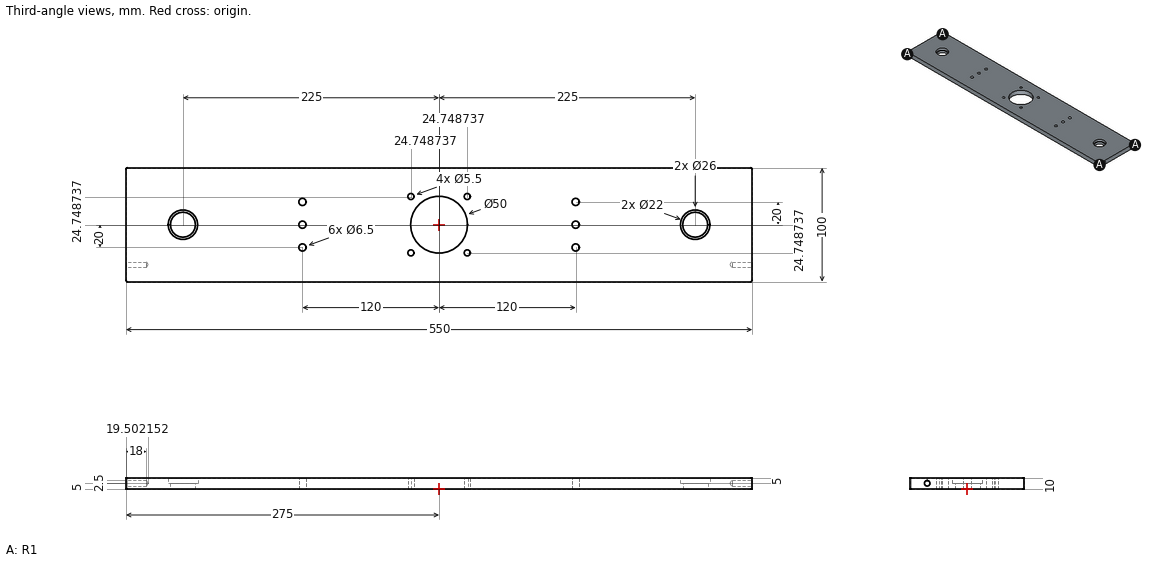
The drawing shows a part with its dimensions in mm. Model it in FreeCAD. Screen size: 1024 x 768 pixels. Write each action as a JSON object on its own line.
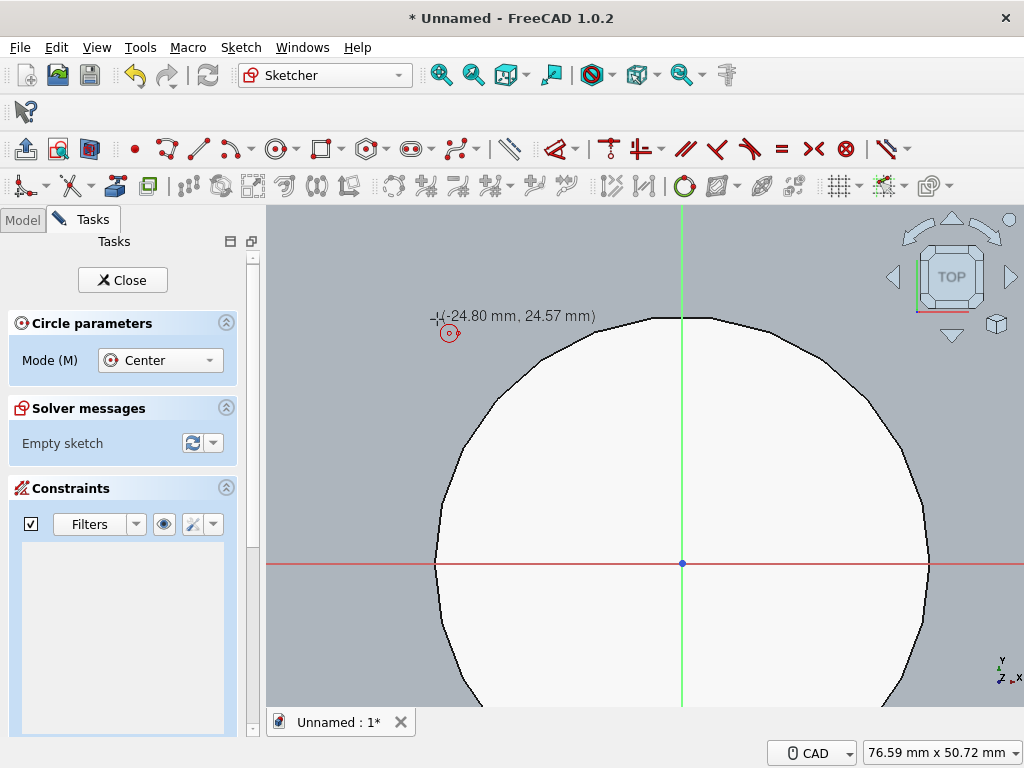
{"action": "left_click", "coordinate": [437, 319]}
{"action": "left_click", "coordinate": [457, 300]}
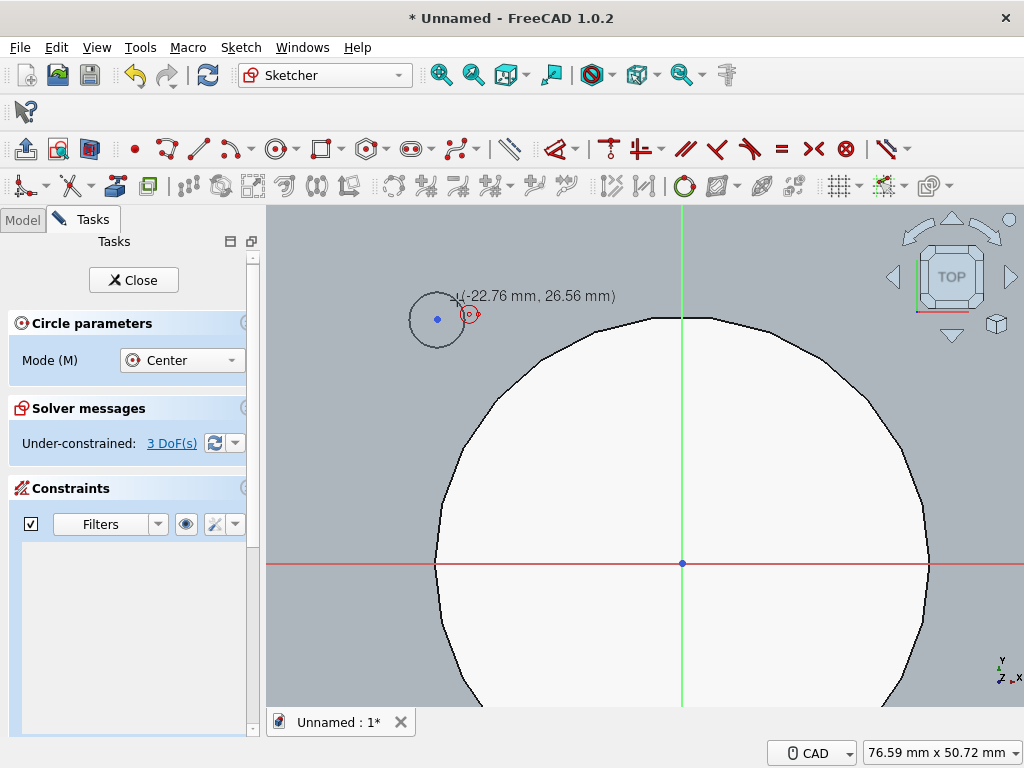
{"action": "scroll", "coordinate": [448, 325], "scroll_direction": "down", "scroll_amount": 3}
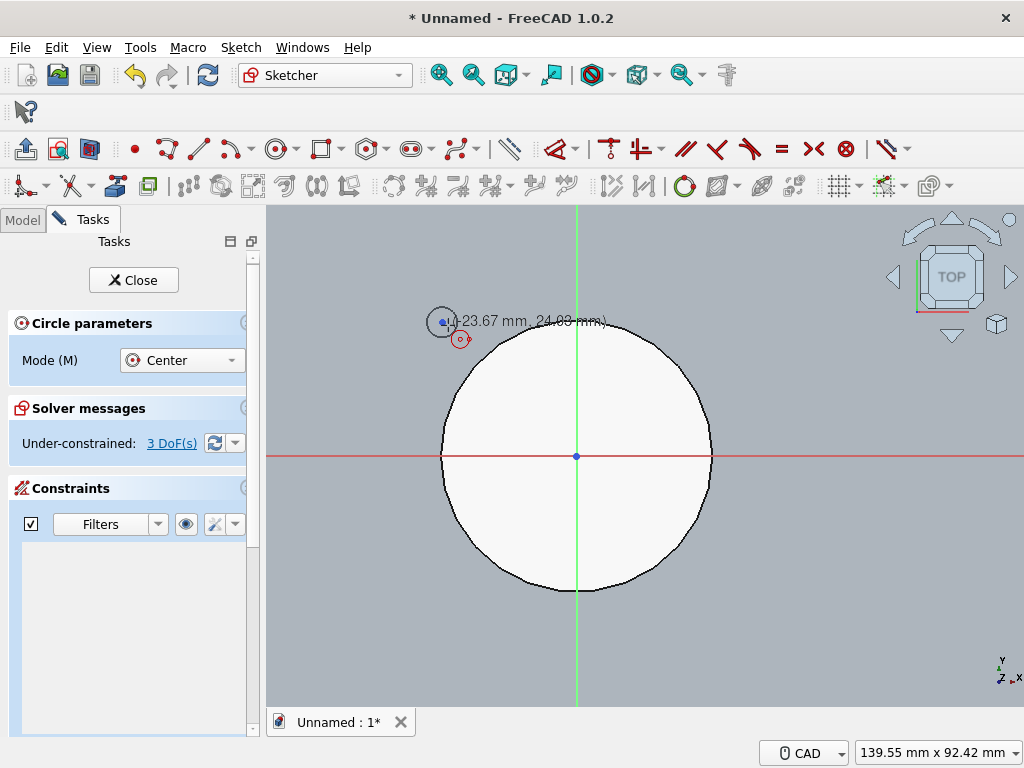
{"action": "scroll", "coordinate": [711, 322], "scroll_direction": "up", "scroll_amount": 3}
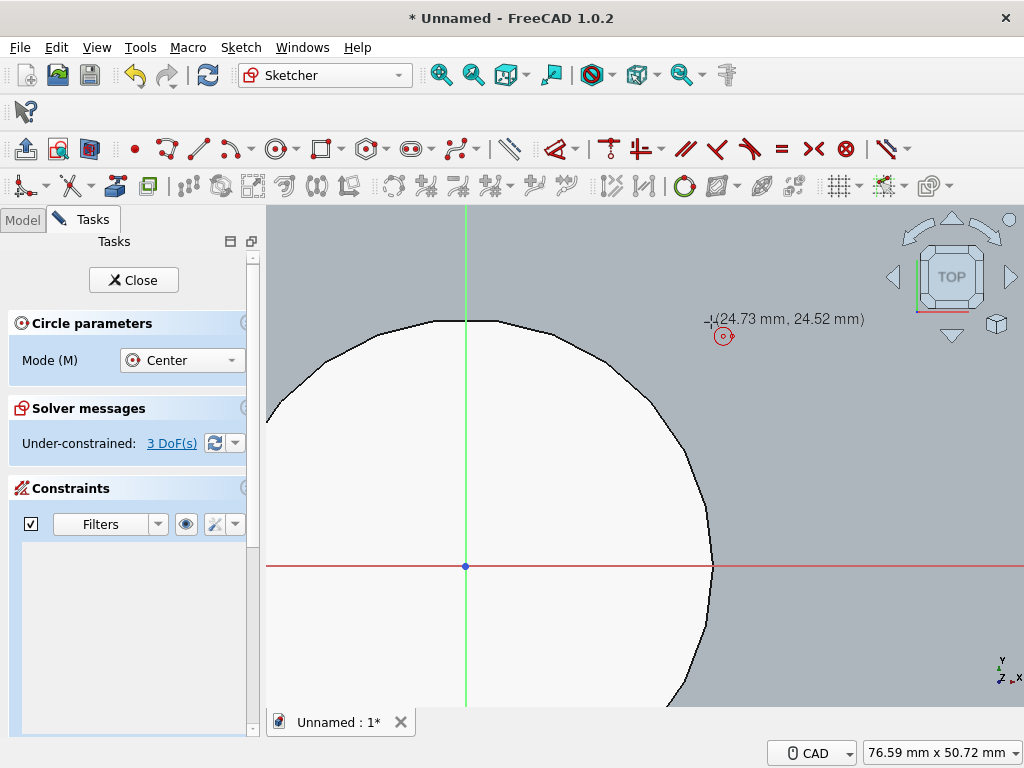
{"action": "left_click", "coordinate": [711, 321]}
{"action": "left_click", "coordinate": [730, 302]}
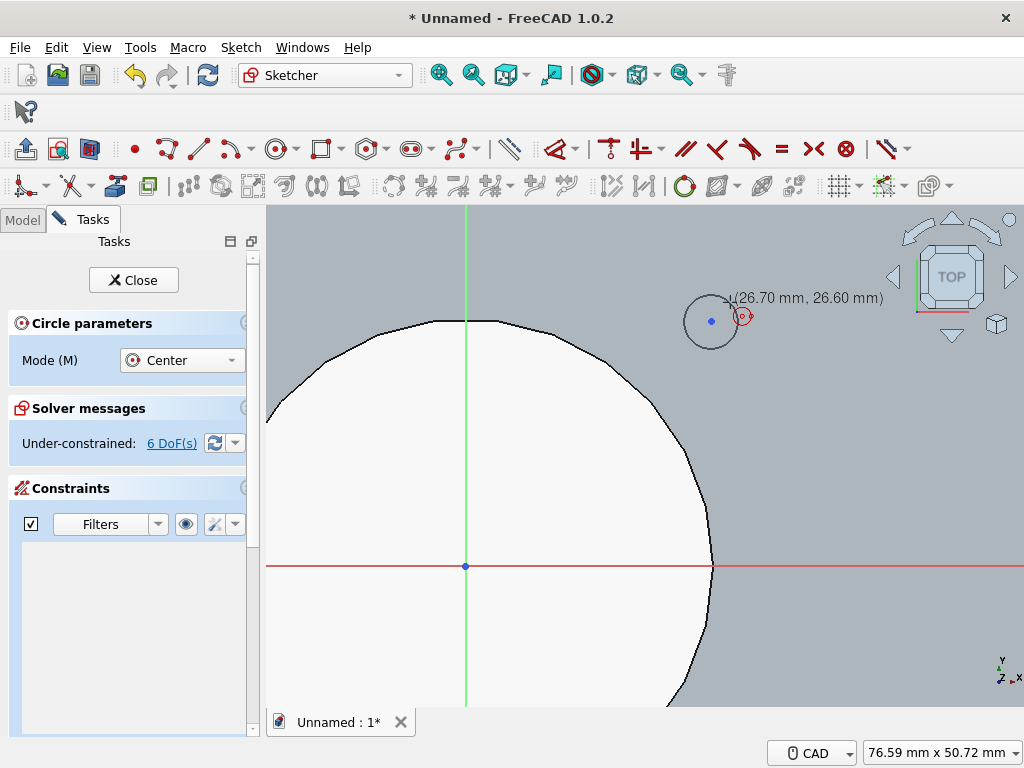
{"action": "scroll", "coordinate": [711, 322], "scroll_direction": "down", "scroll_amount": 3}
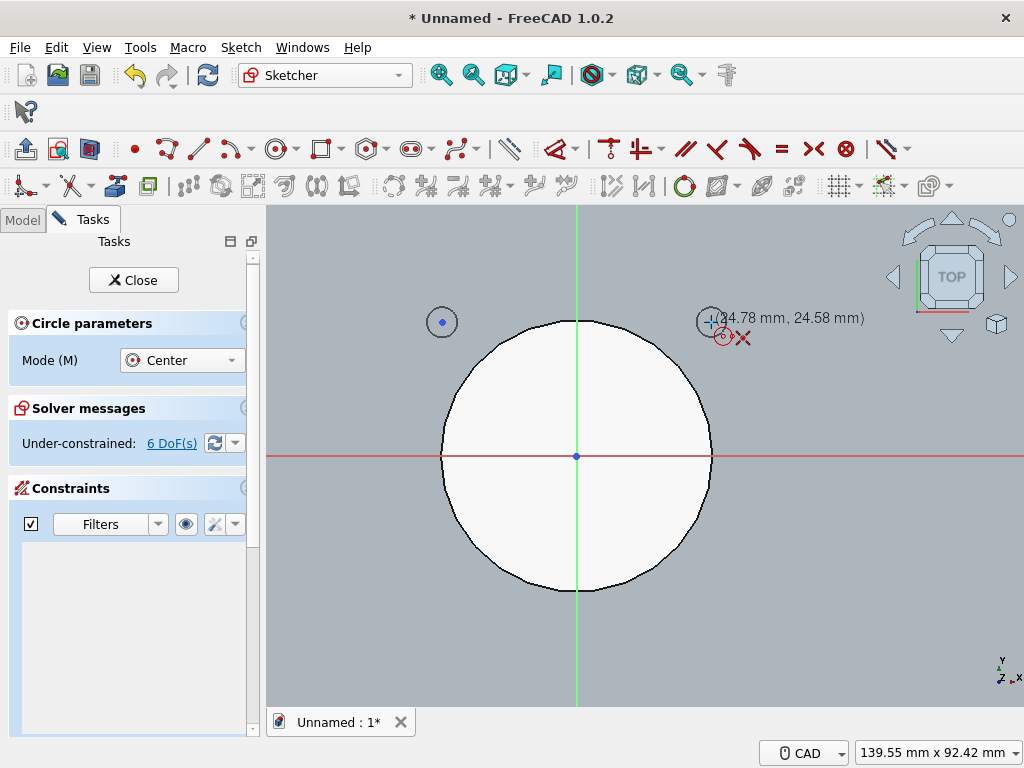
{"action": "scroll", "coordinate": [711, 591], "scroll_direction": "up", "scroll_amount": 3}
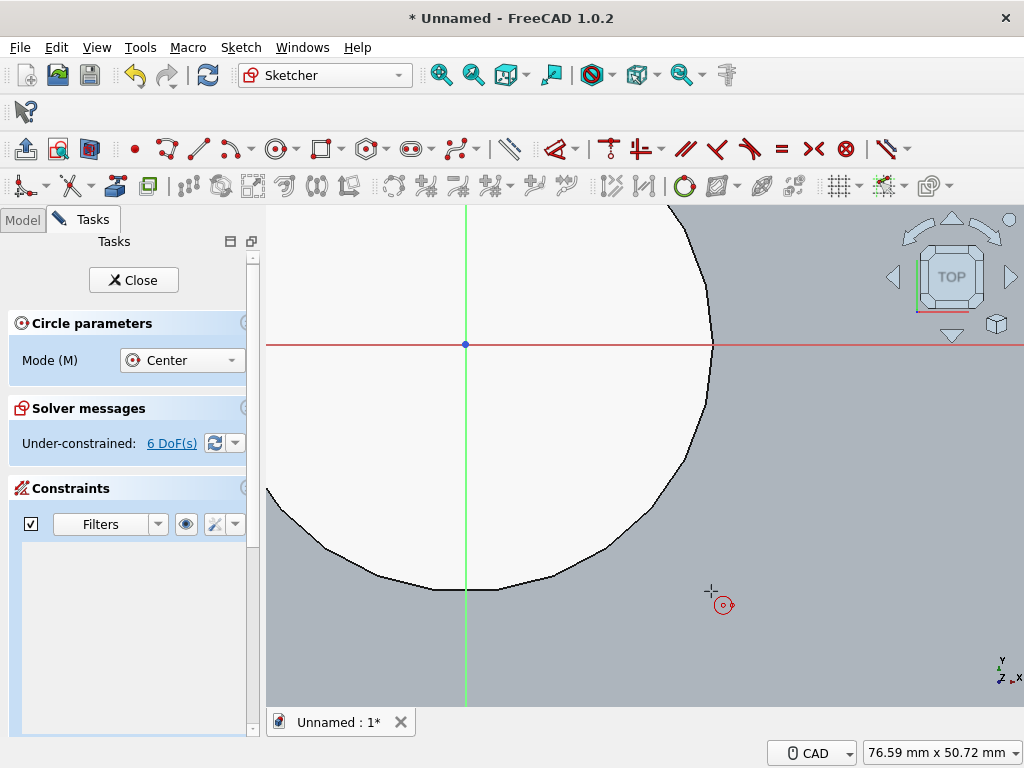
{"action": "left_click", "coordinate": [711, 590]}
{"action": "left_click", "coordinate": [730, 570]}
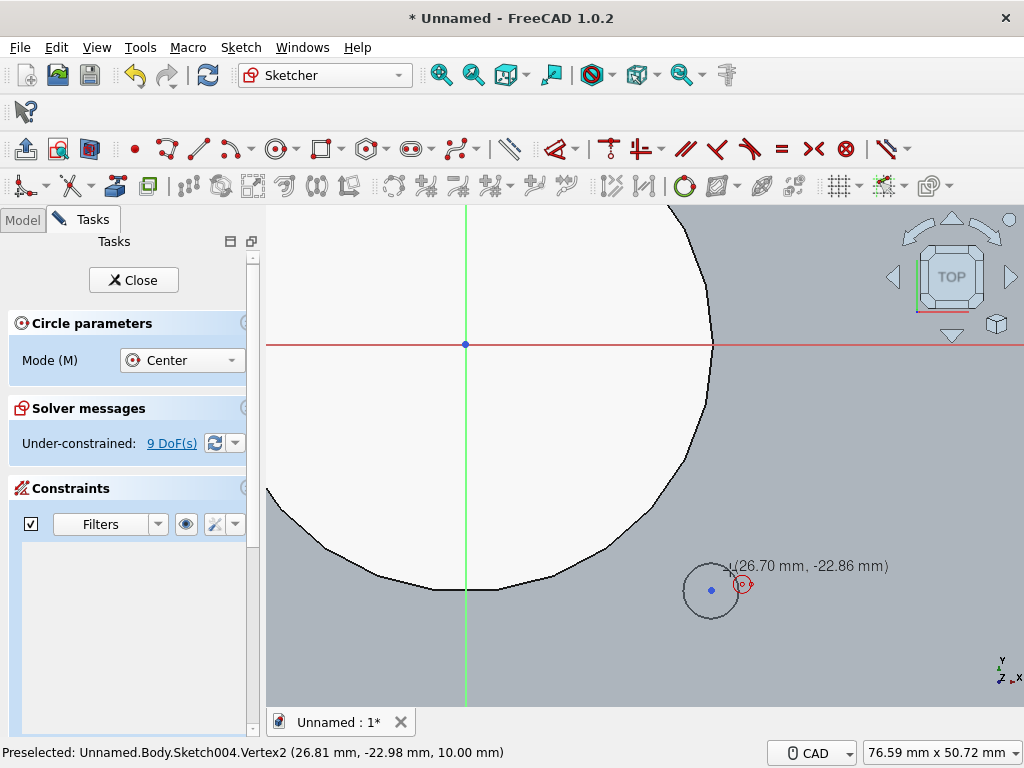
{"action": "scroll", "coordinate": [711, 591], "scroll_direction": "down", "scroll_amount": 3}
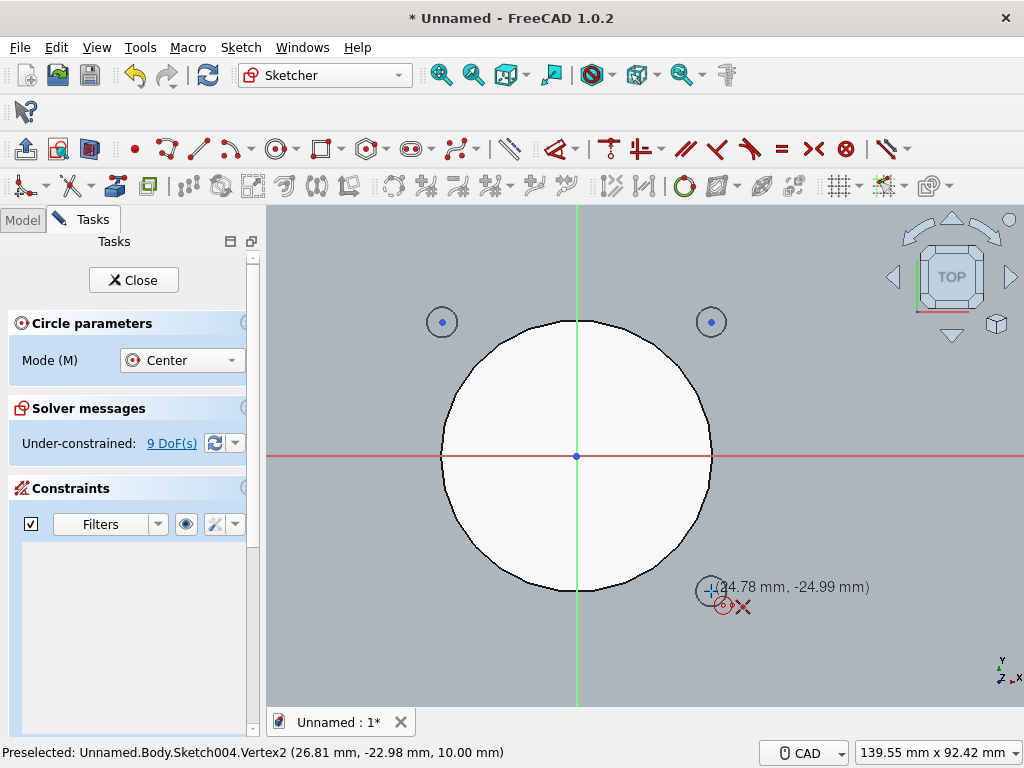
{"action": "scroll", "coordinate": [442, 591], "scroll_direction": "up", "scroll_amount": 3}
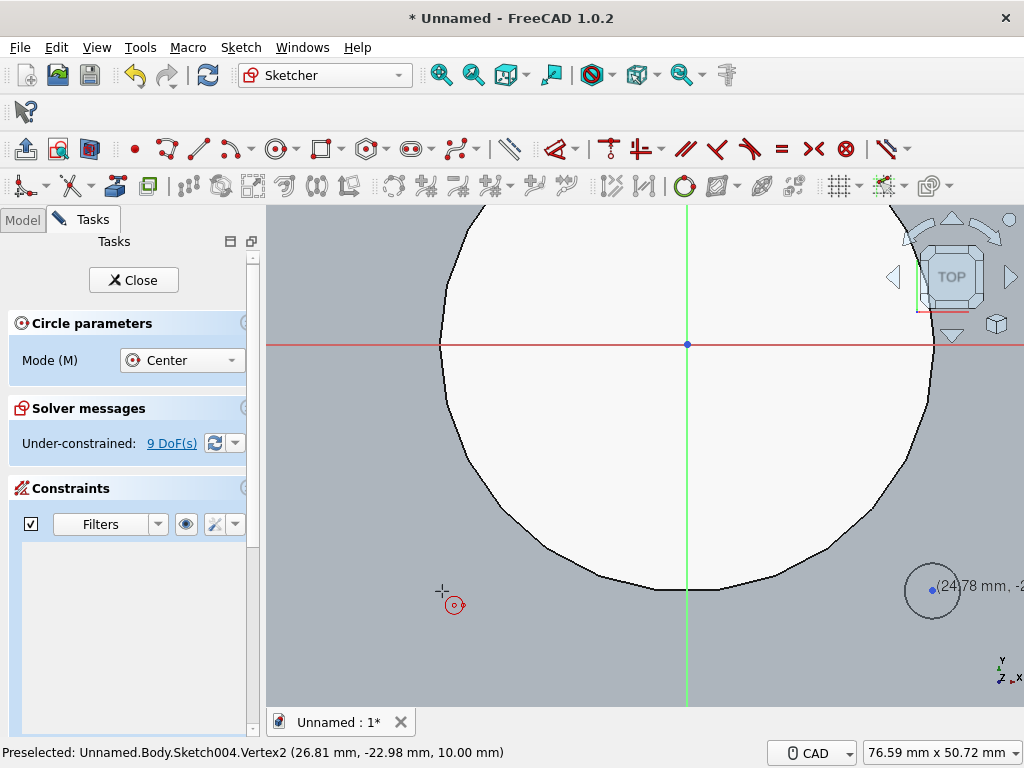
{"action": "left_click", "coordinate": [442, 590]}
{"action": "left_click", "coordinate": [461, 570]}
{"action": "key", "text": "Escape"}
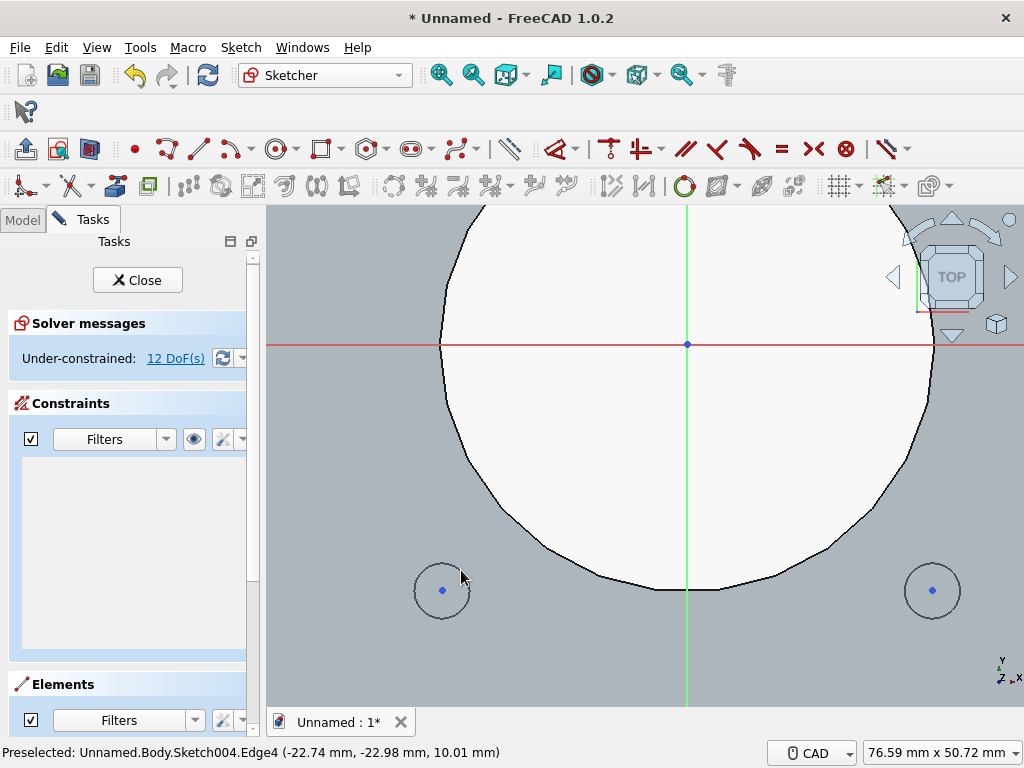
{"action": "scroll", "coordinate": [442, 591], "scroll_direction": "down", "scroll_amount": 3}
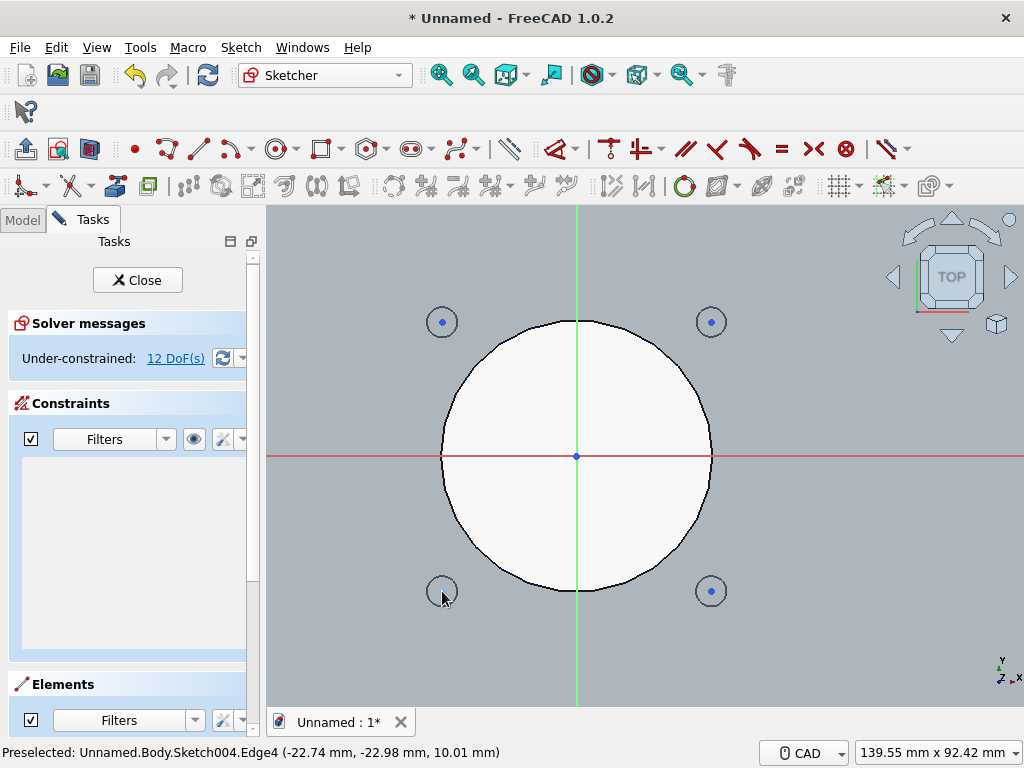
{"action": "left_click", "coordinate": [453, 312]}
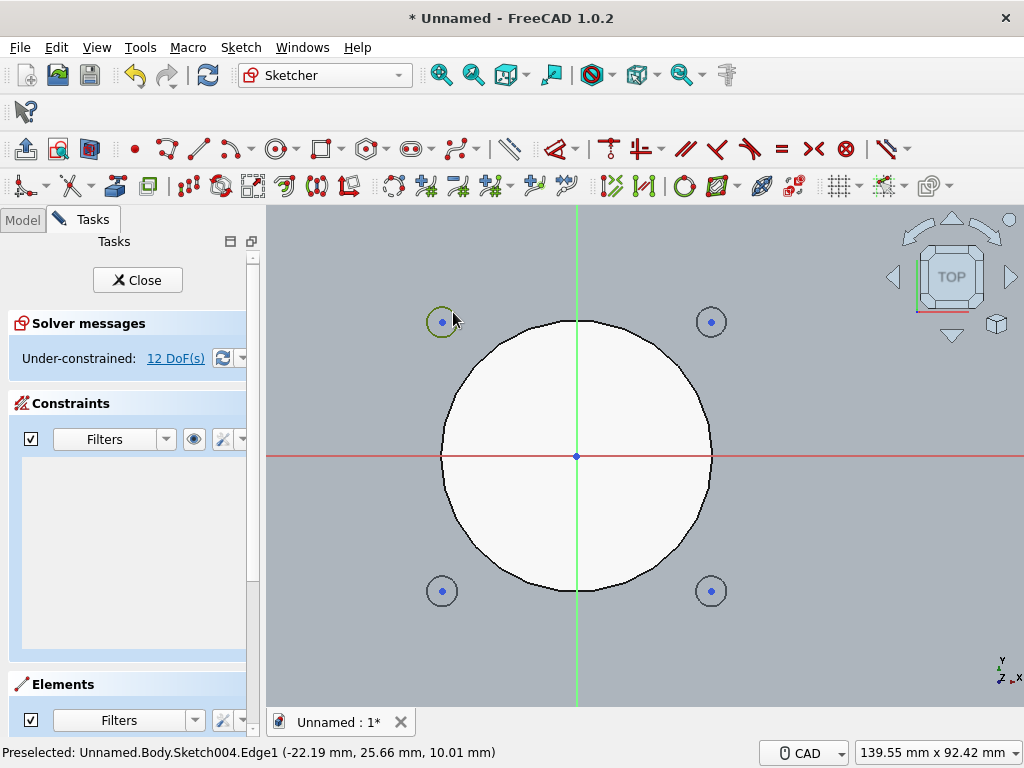
{"action": "left_click", "coordinate": [722, 312]}